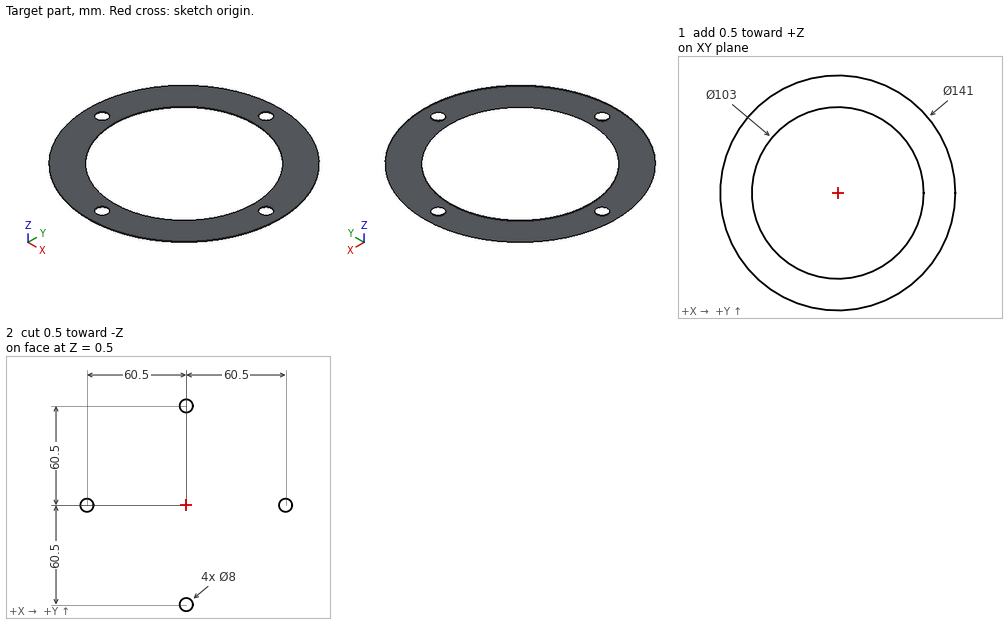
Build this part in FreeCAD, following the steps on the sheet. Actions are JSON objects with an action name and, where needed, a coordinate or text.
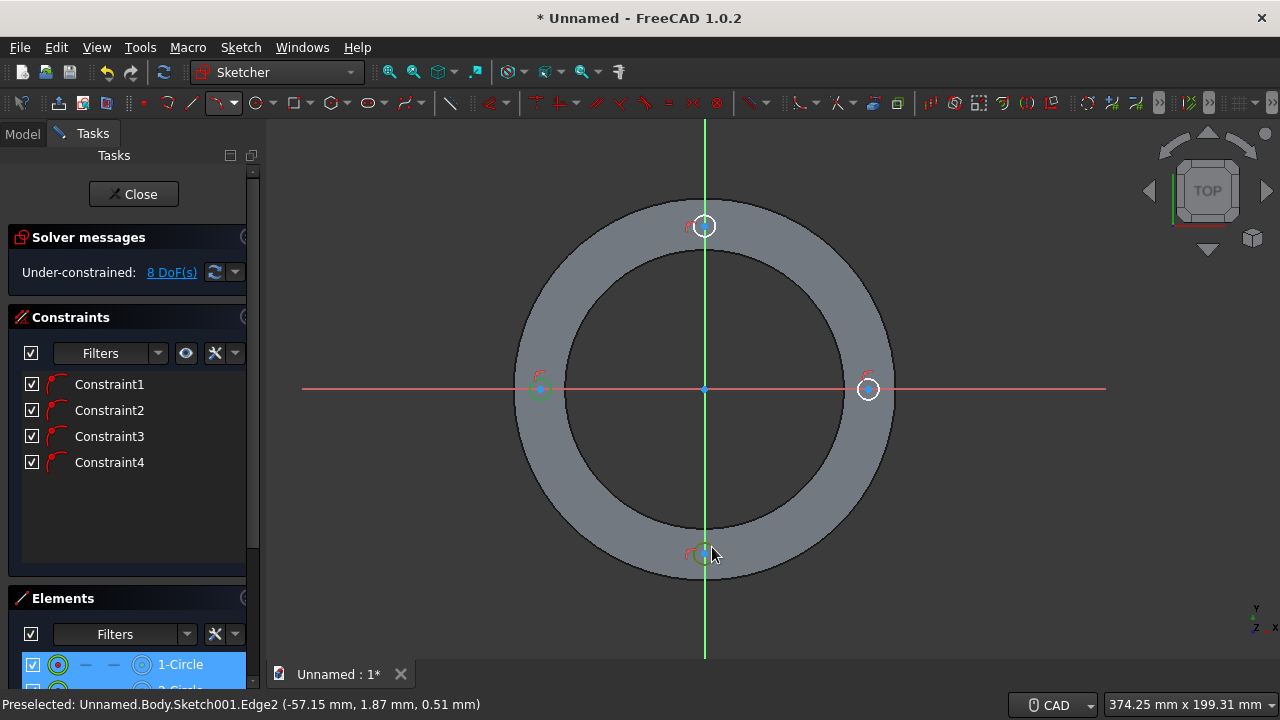
{"action": "scroll", "coordinate": [712, 218], "scroll_direction": "up", "scroll_amount": 4}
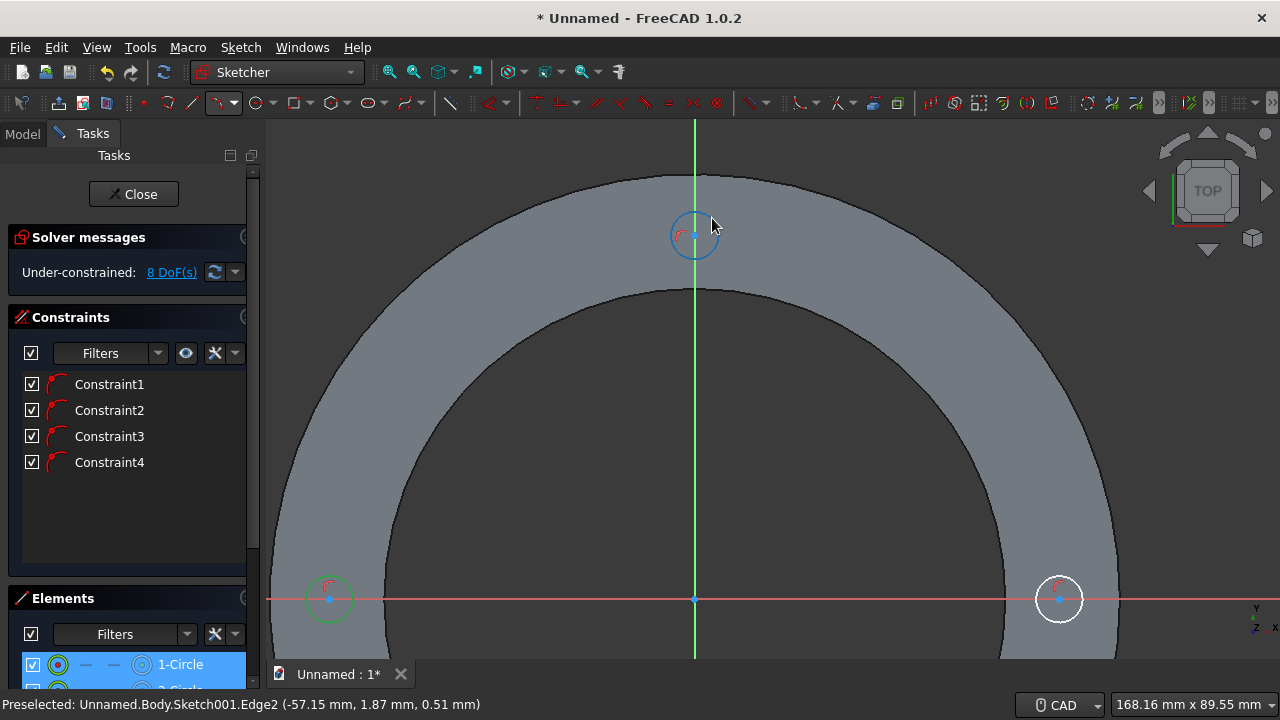
{"action": "left_click", "coordinate": [712, 219]}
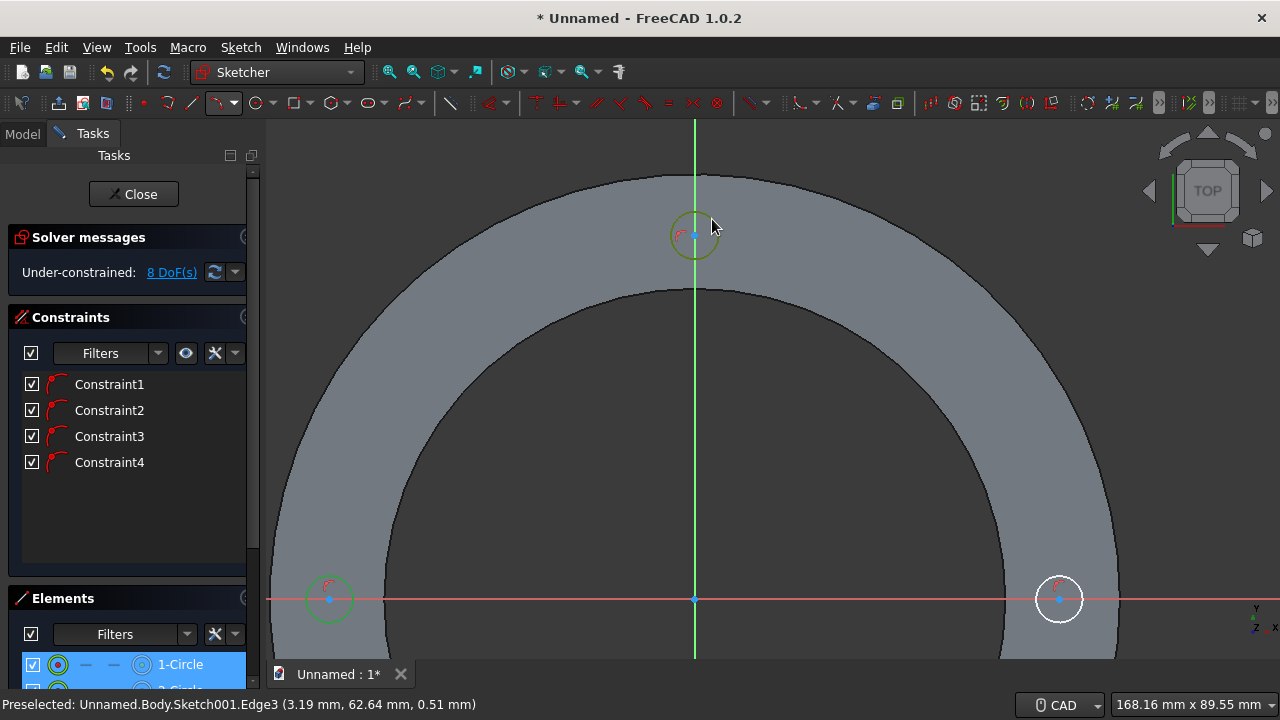
{"action": "left_click", "coordinate": [1076, 583]}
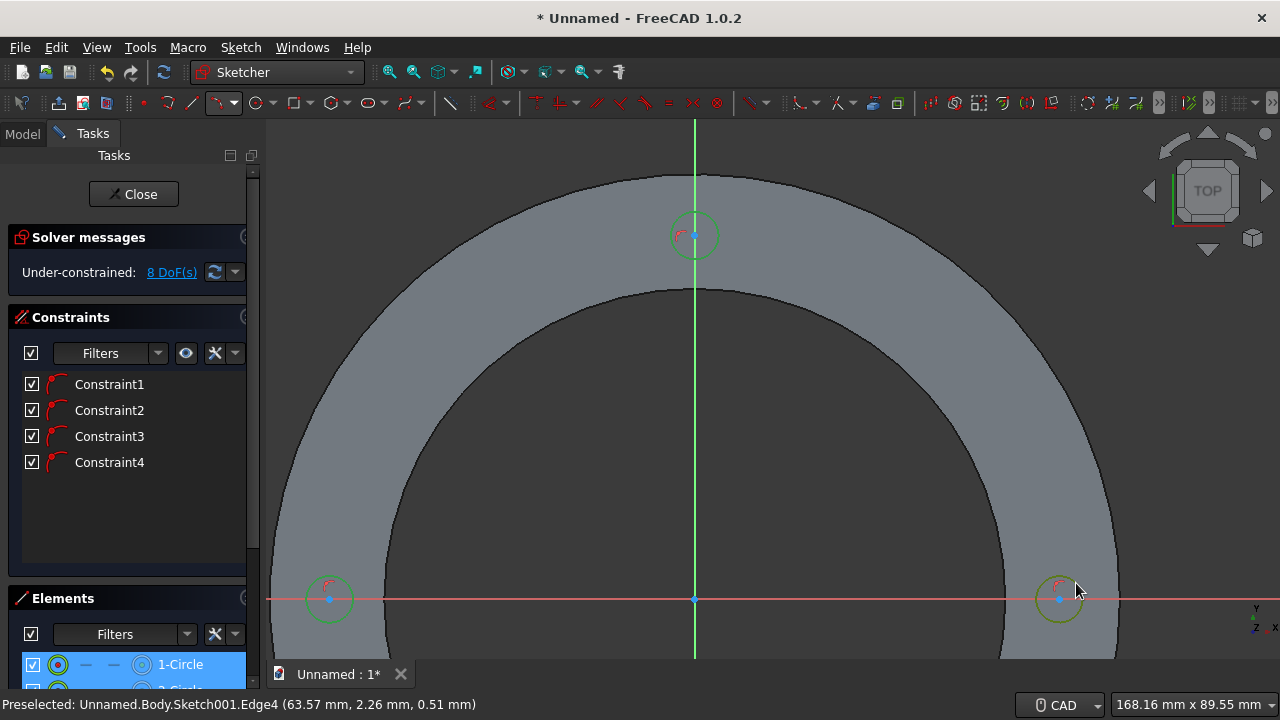
{"action": "left_click", "coordinate": [670, 104]}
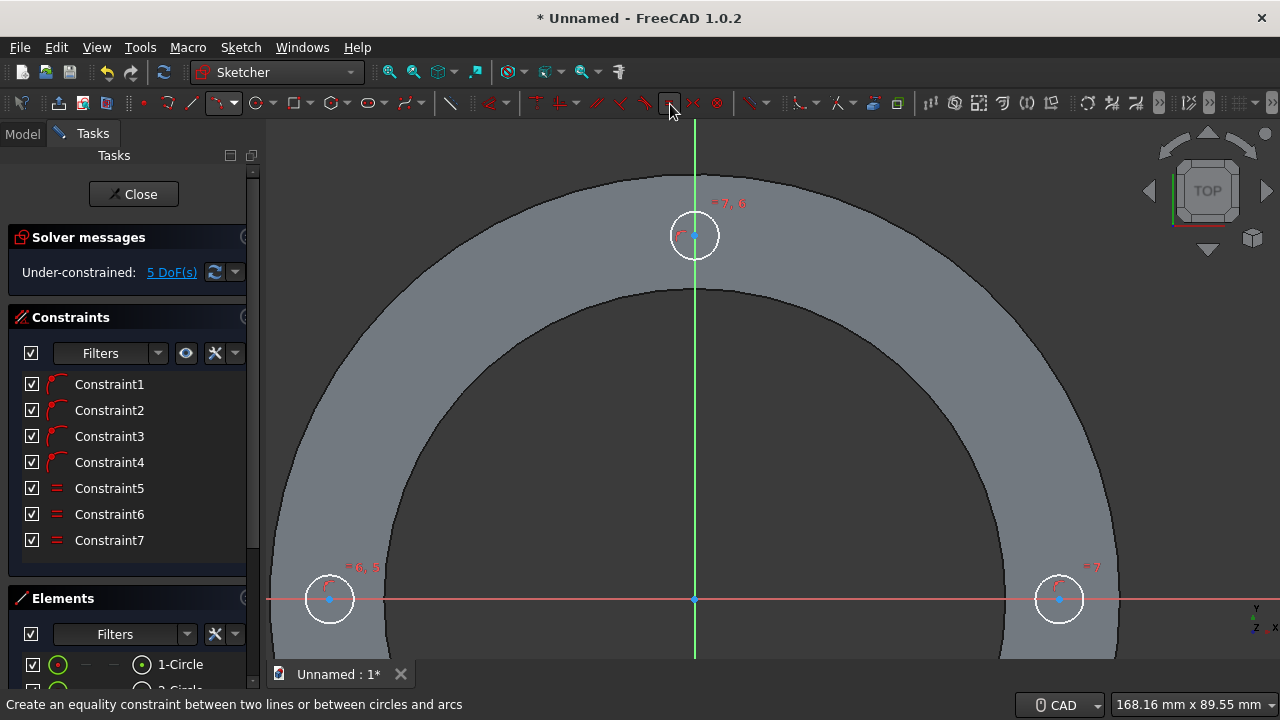
{"action": "left_click", "coordinate": [490, 104]}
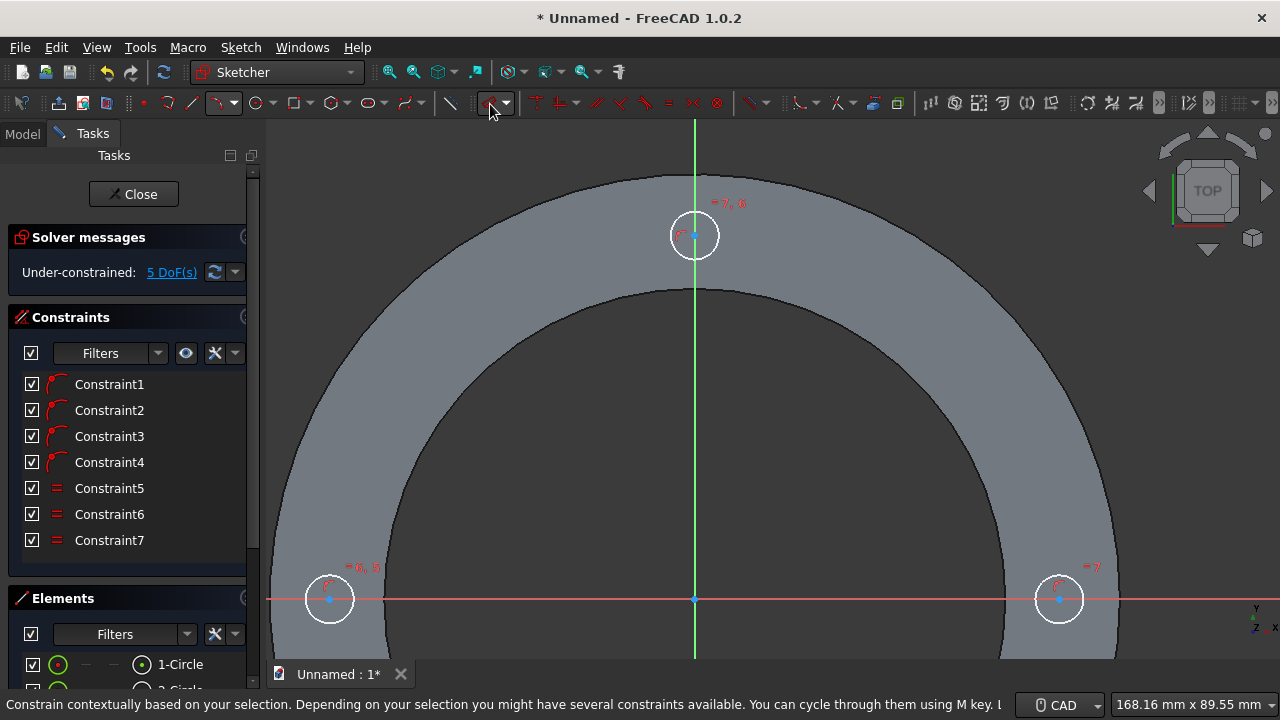
{"action": "scroll", "coordinate": [712, 217], "scroll_direction": "down", "scroll_amount": 4}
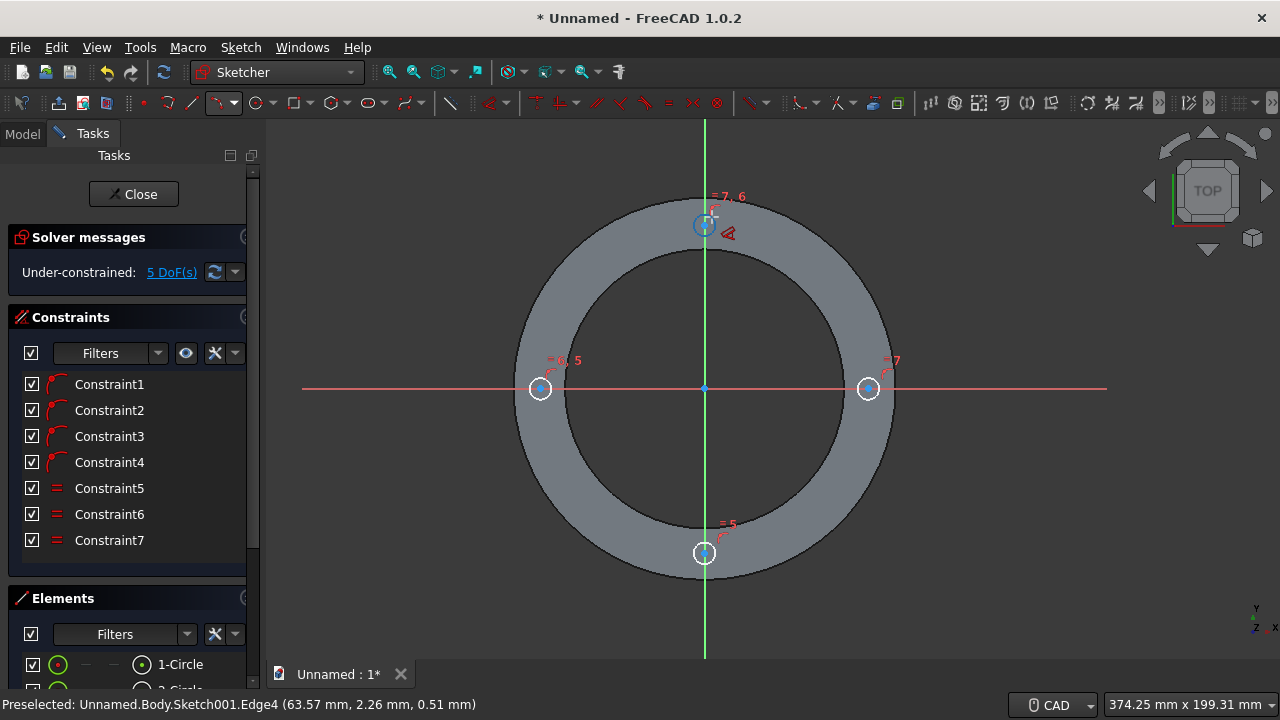
{"action": "scroll", "coordinate": [712, 546], "scroll_direction": "up", "scroll_amount": 4}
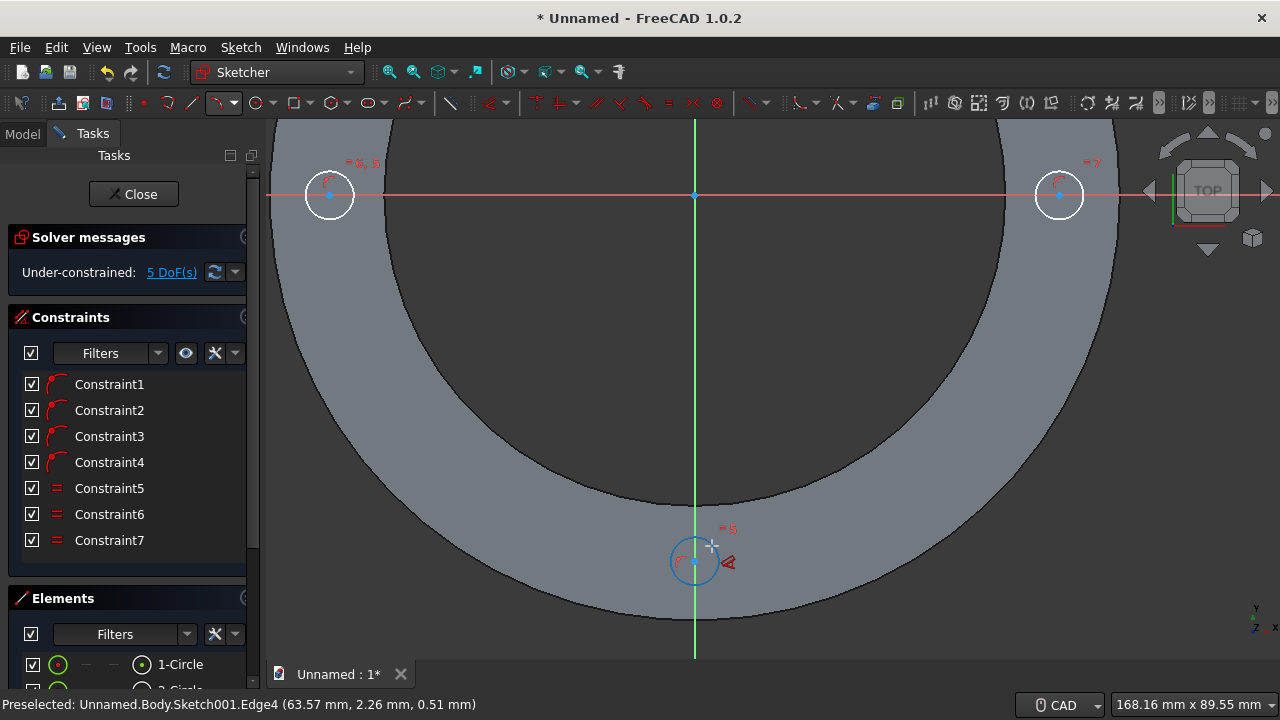
{"action": "left_click", "coordinate": [712, 544]}
{"action": "left_click", "coordinate": [735, 521]}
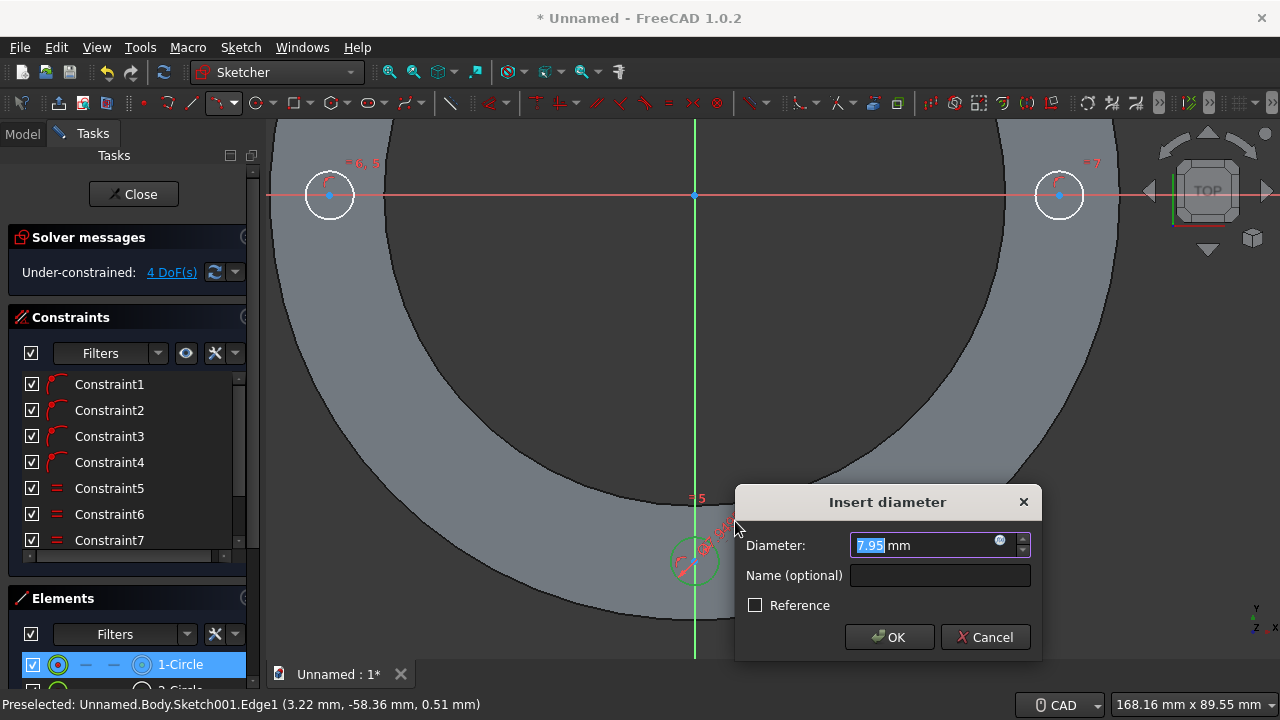
{"action": "type", "text": "8"}
{"action": "key", "text": "Return"}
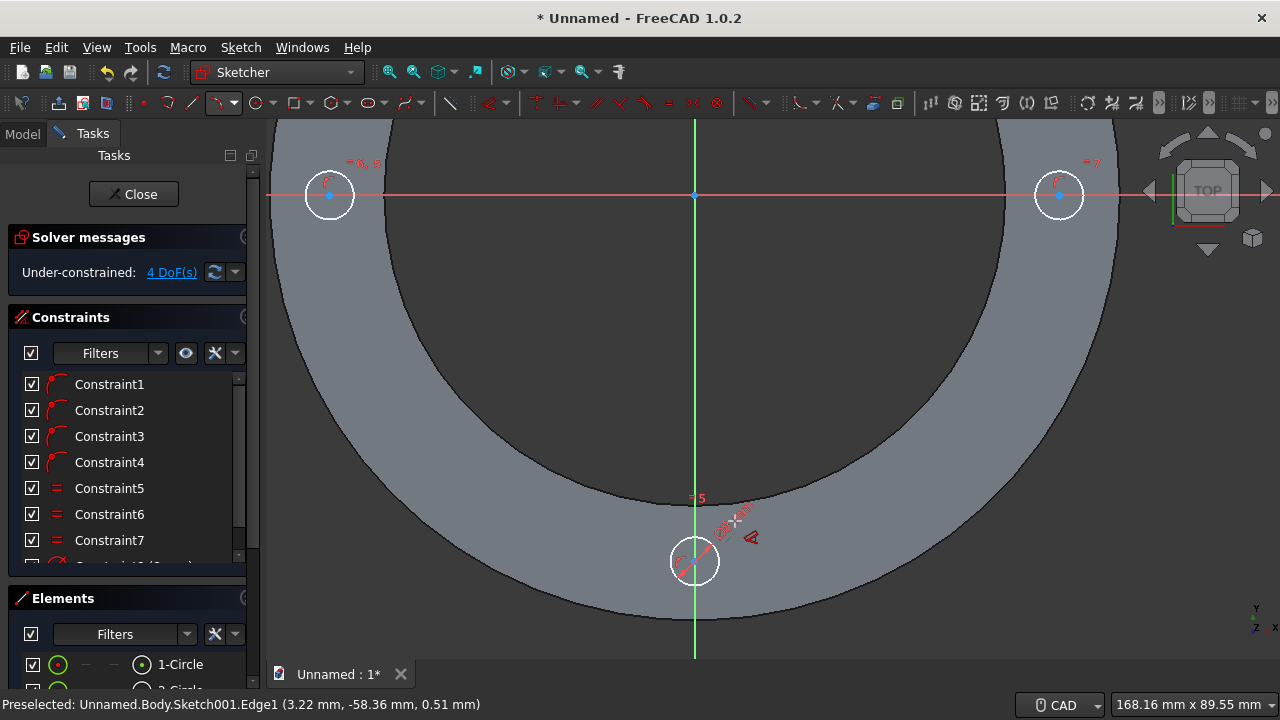
{"action": "left_click", "coordinate": [695, 561]}
{"action": "left_click", "coordinate": [729, 378]}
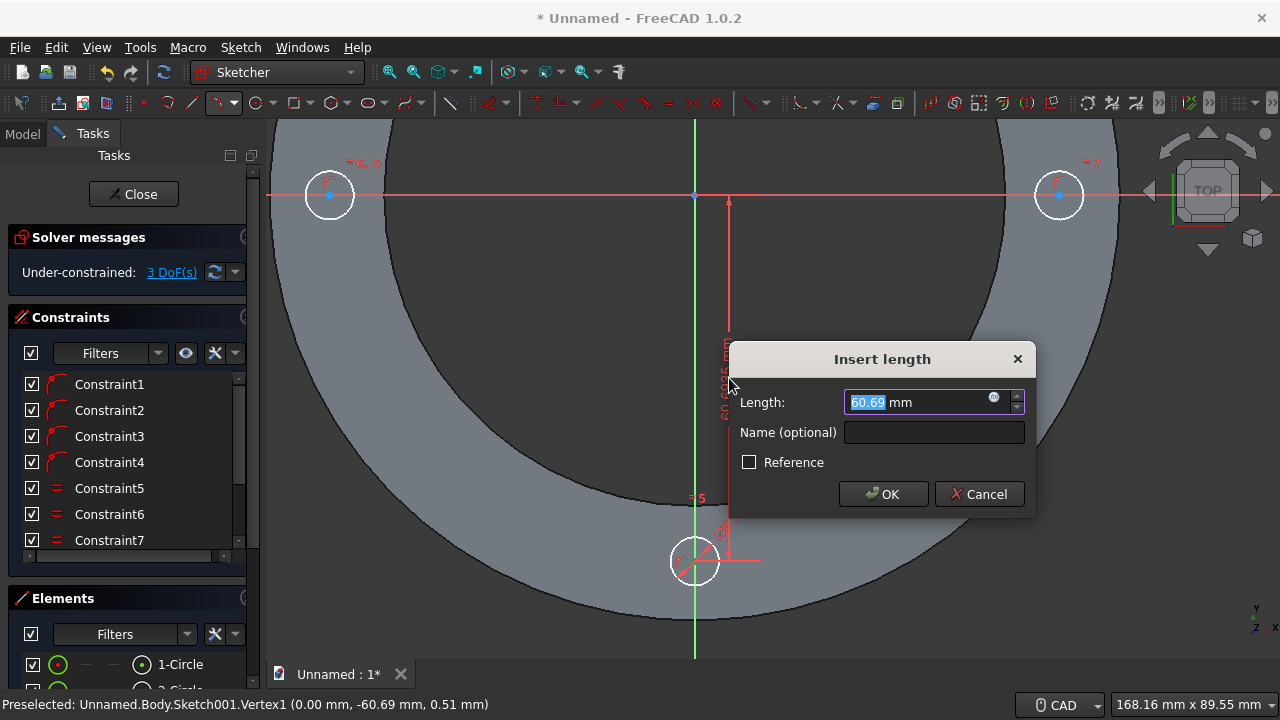
{"action": "type", "text": "60.5"}
{"action": "key", "text": "Return"}